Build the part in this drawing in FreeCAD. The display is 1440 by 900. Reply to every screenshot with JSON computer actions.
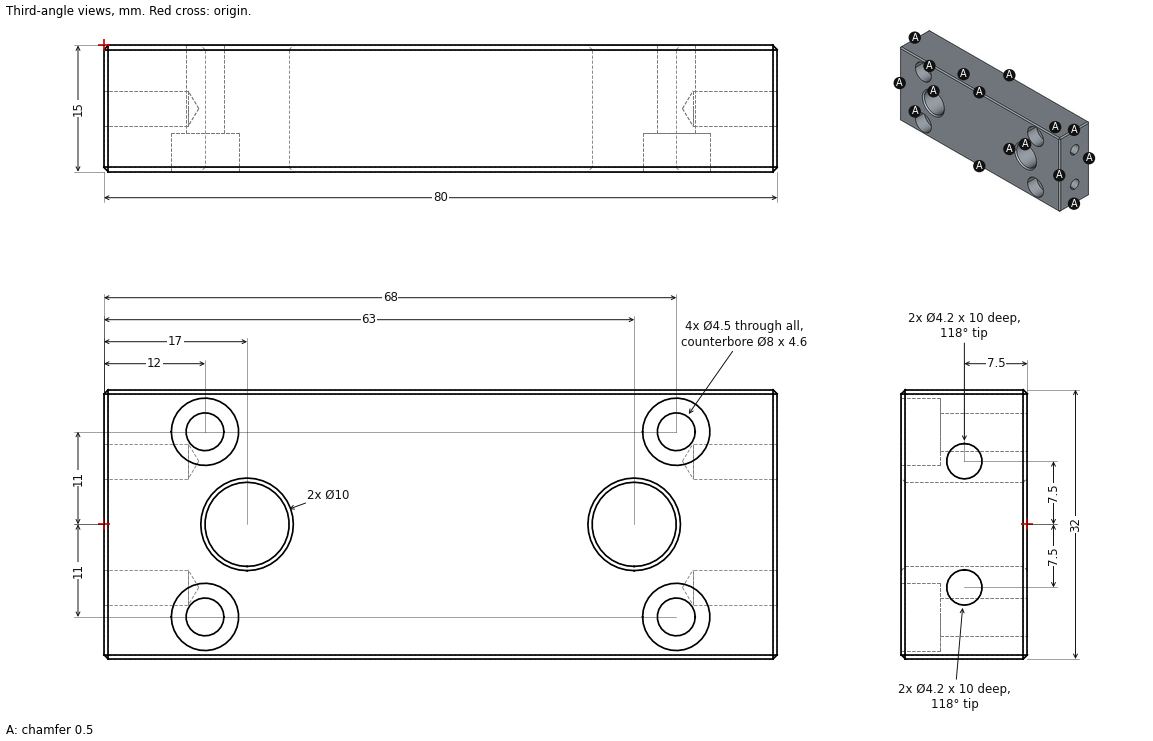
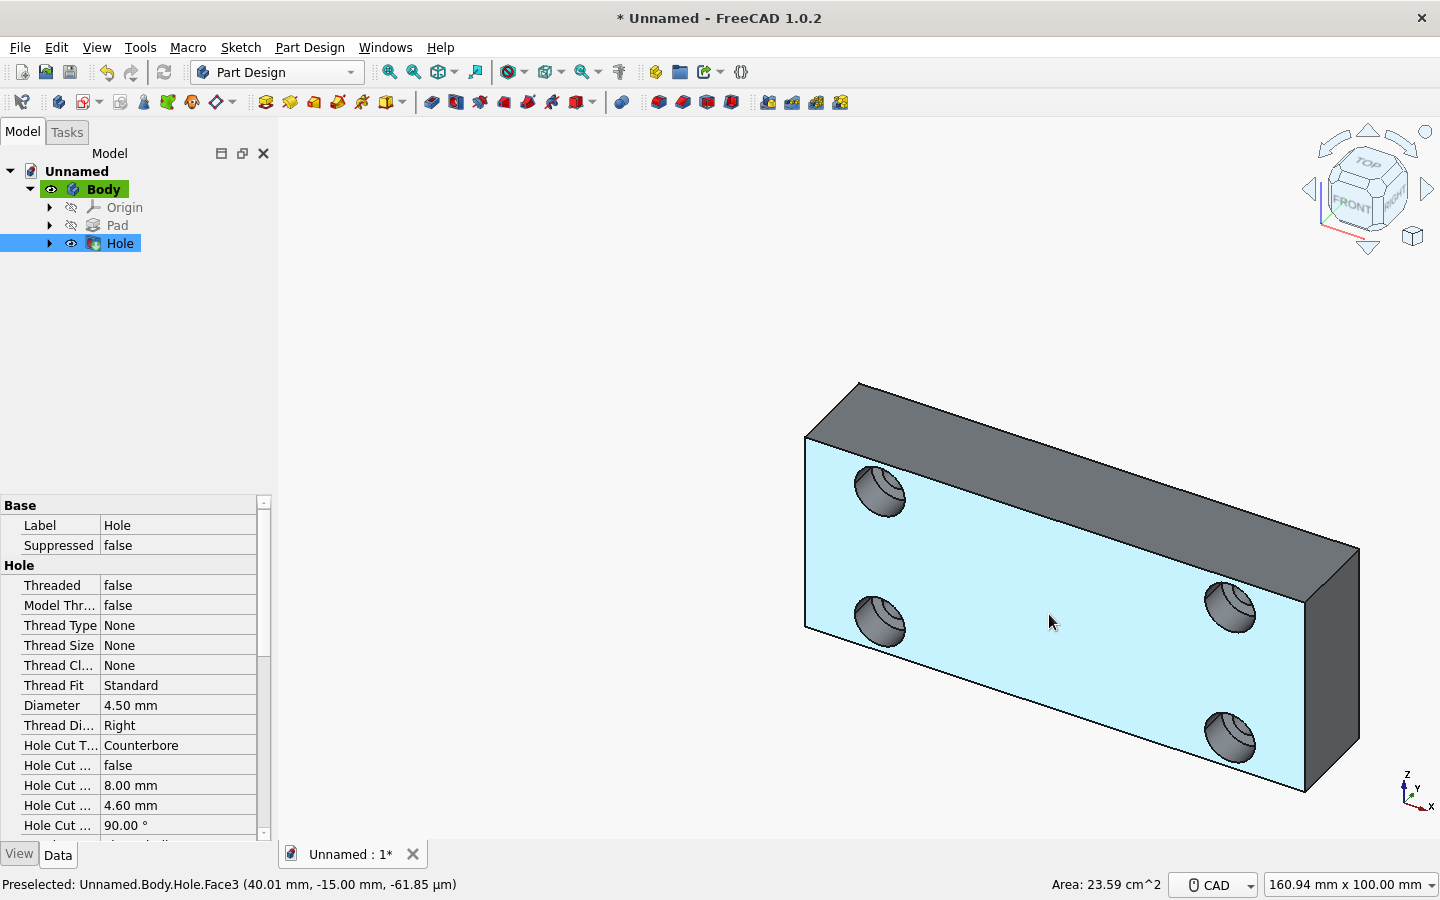
{"action": "left_click", "coordinate": [84, 102]}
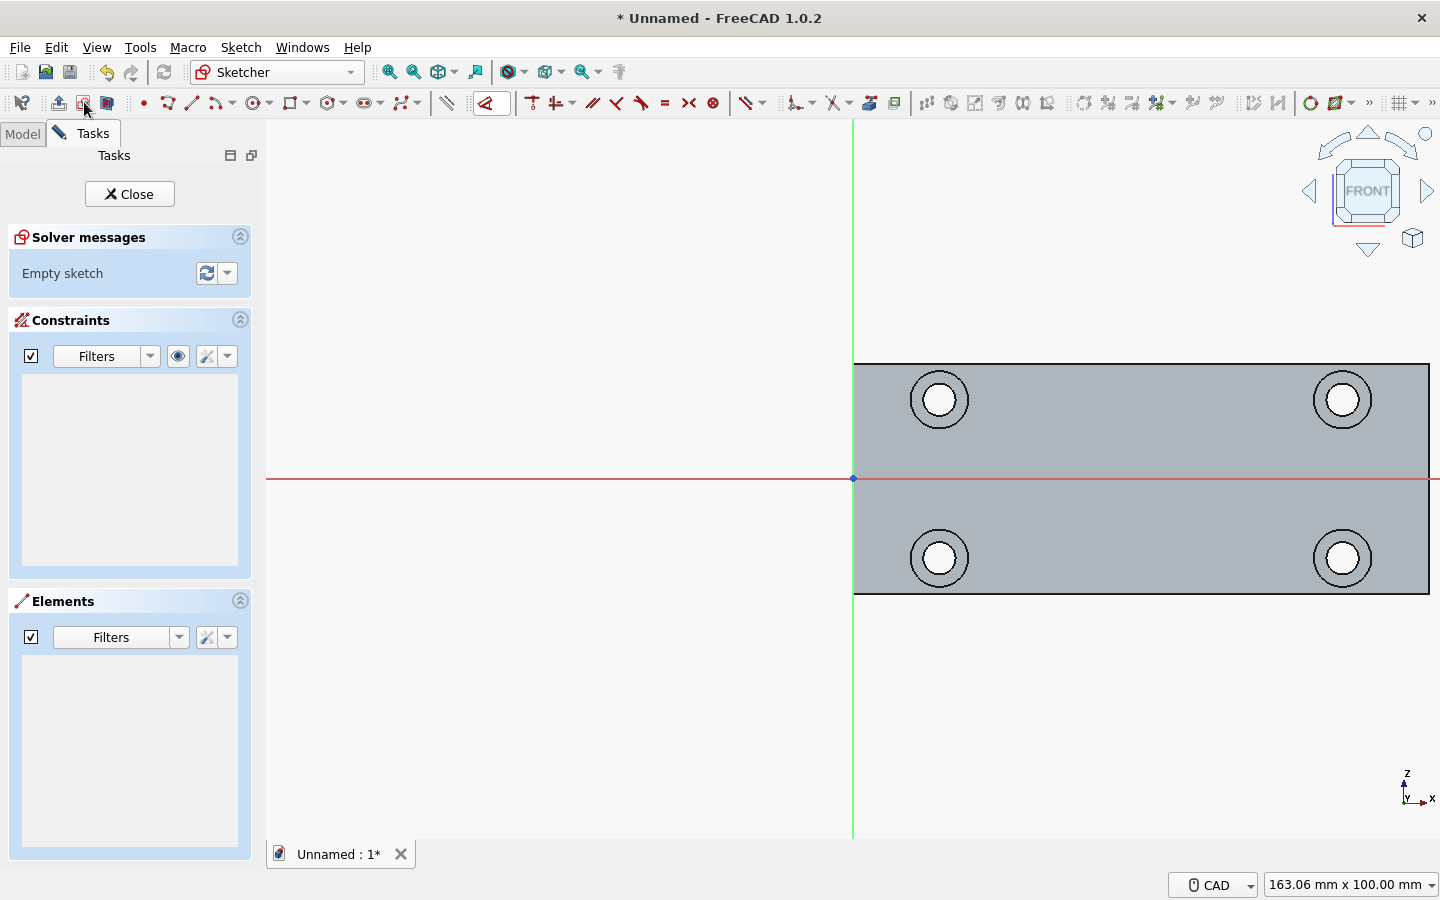
{"action": "scroll", "coordinate": [294, 479], "scroll_direction": "down", "scroll_amount": 1}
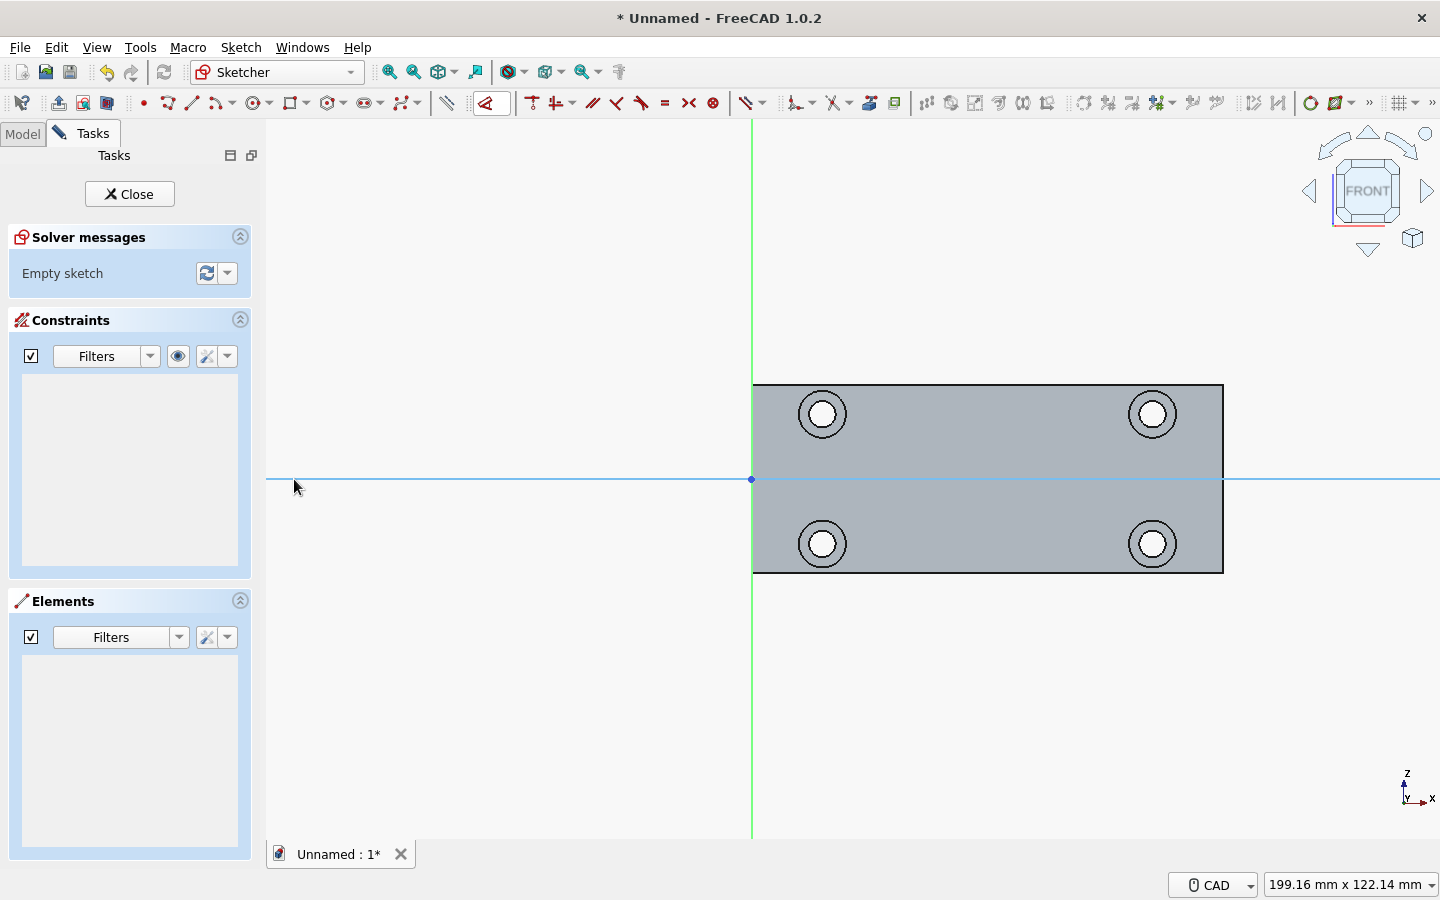
{"action": "scroll", "coordinate": [1156, 479], "scroll_direction": "up", "scroll_amount": 3}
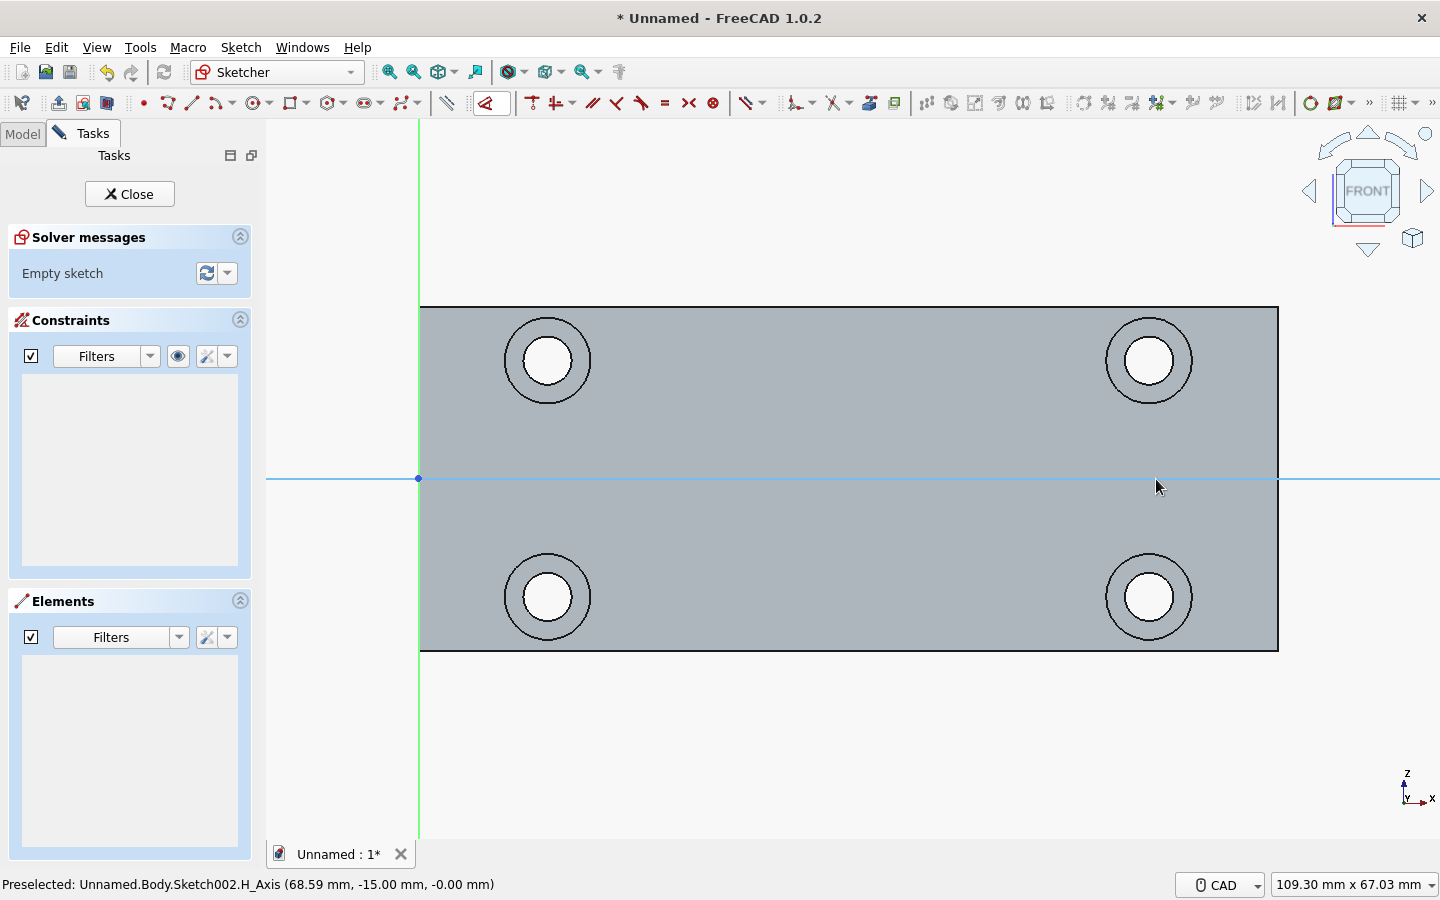
{"action": "left_click", "coordinate": [254, 104]}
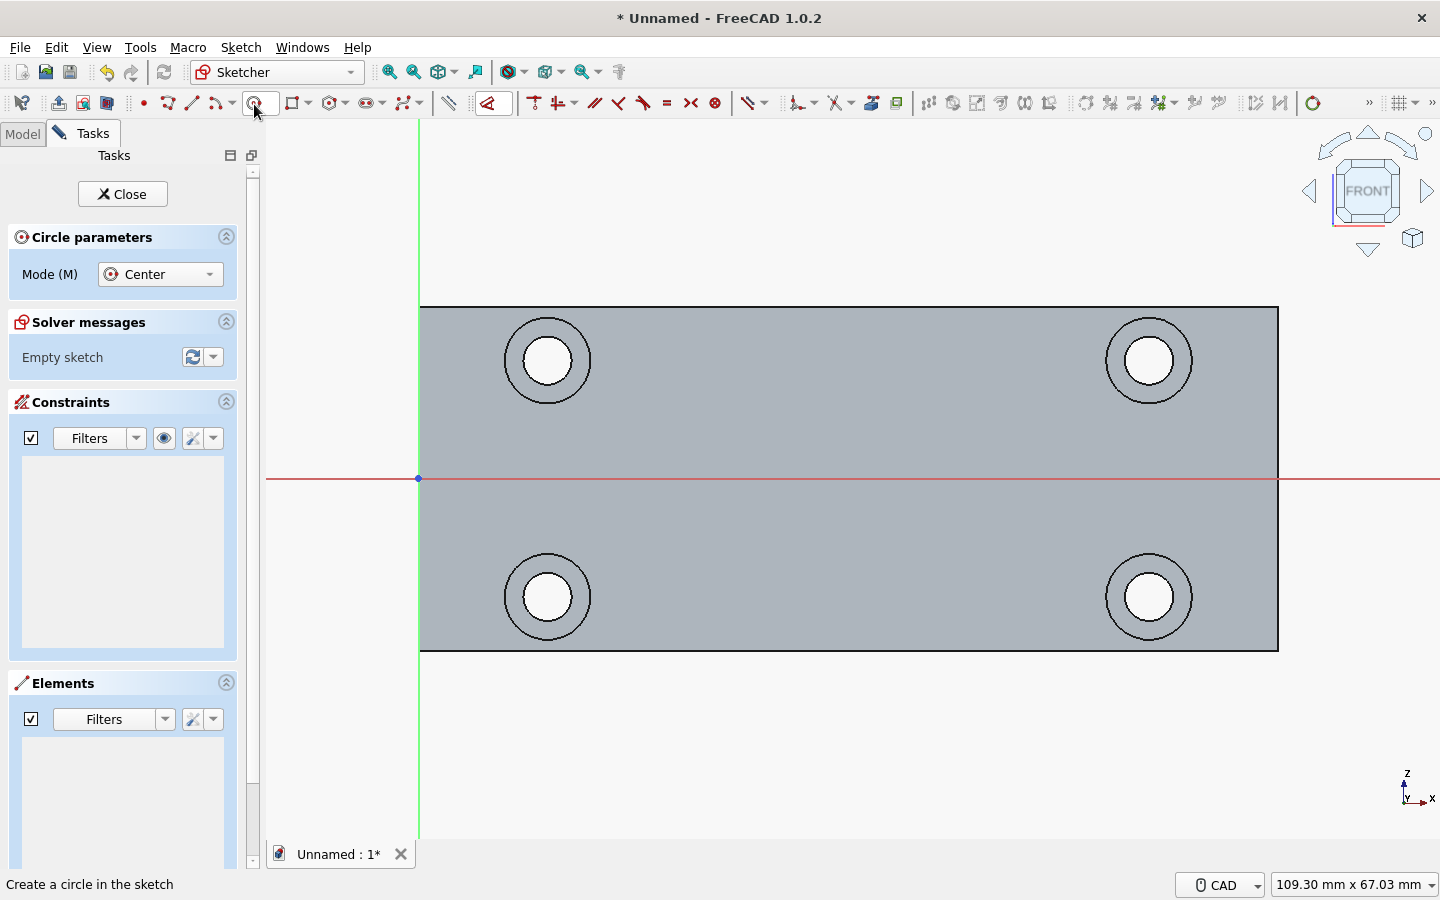
{"action": "left_click", "coordinate": [601, 479]}
{"action": "left_click", "coordinate": [639, 441]}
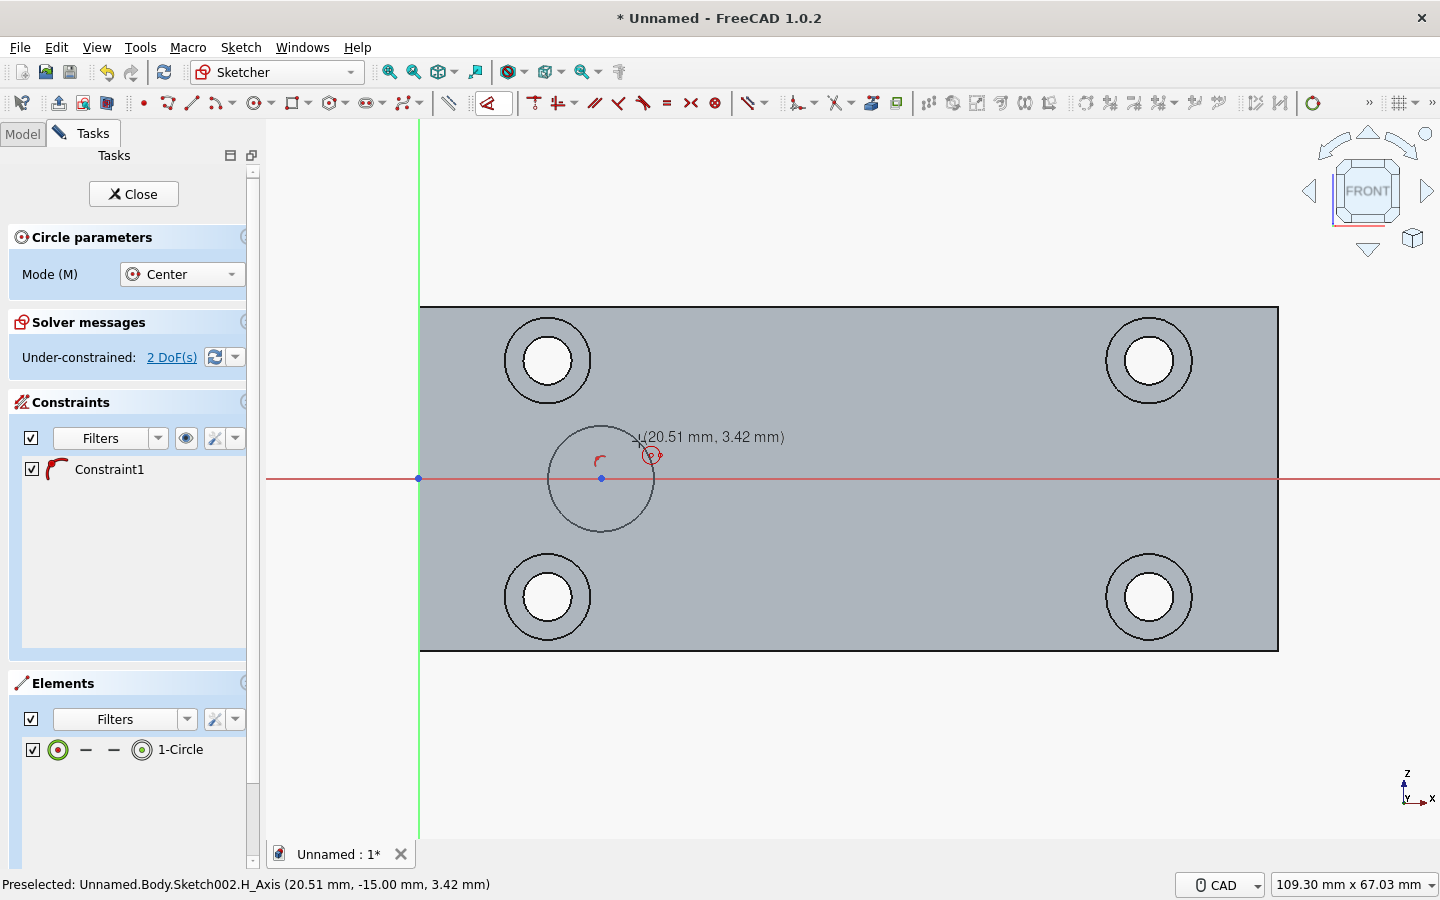
{"action": "left_click", "coordinate": [1095, 479]}
{"action": "left_click", "coordinate": [1133, 441]}
{"action": "key", "text": "Escape"}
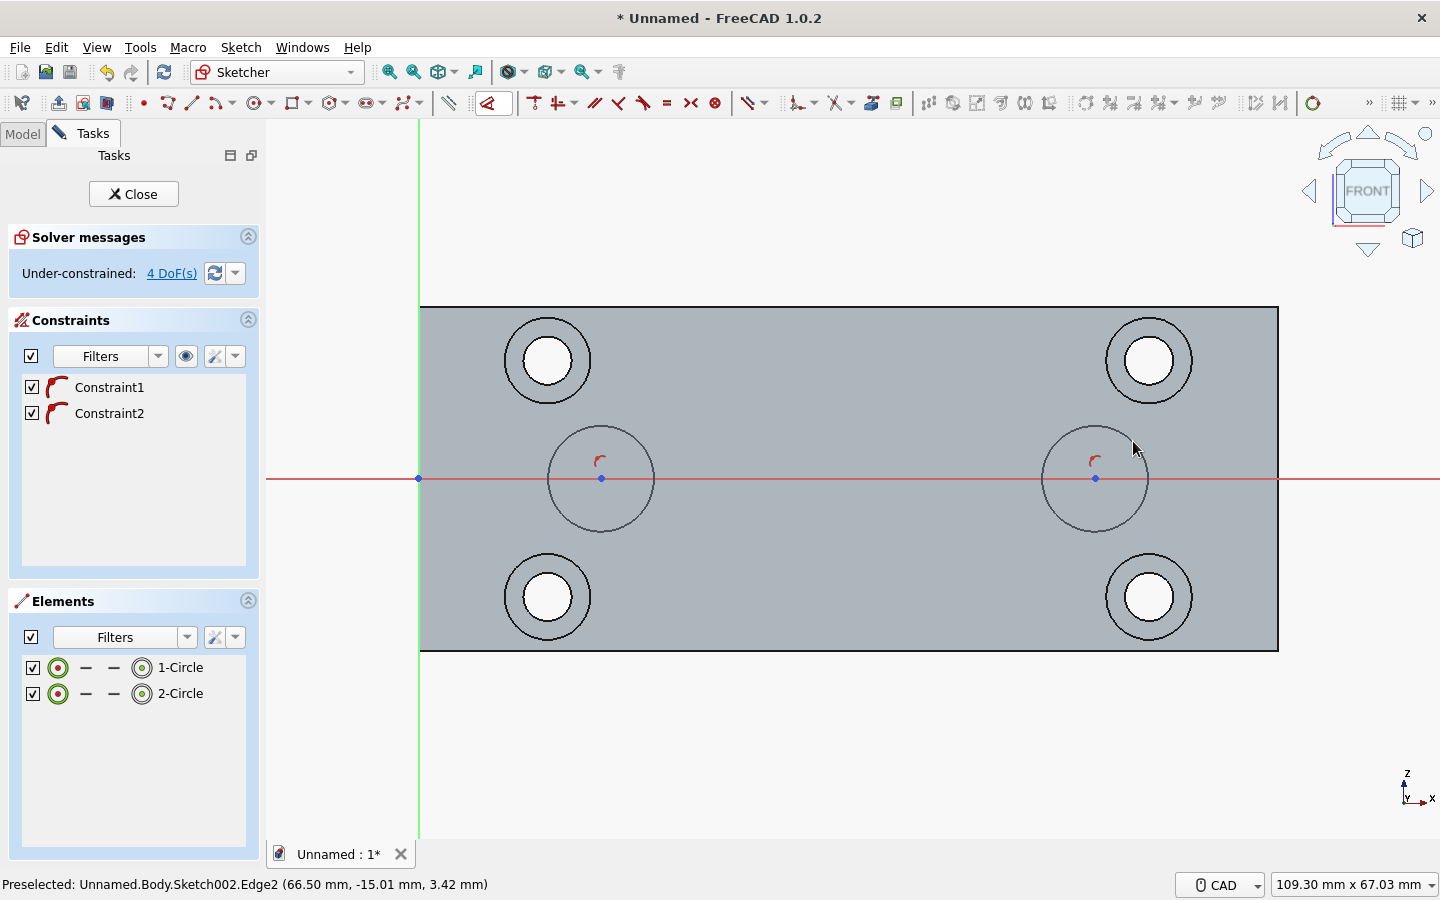
{"action": "left_click", "coordinate": [638, 441]}